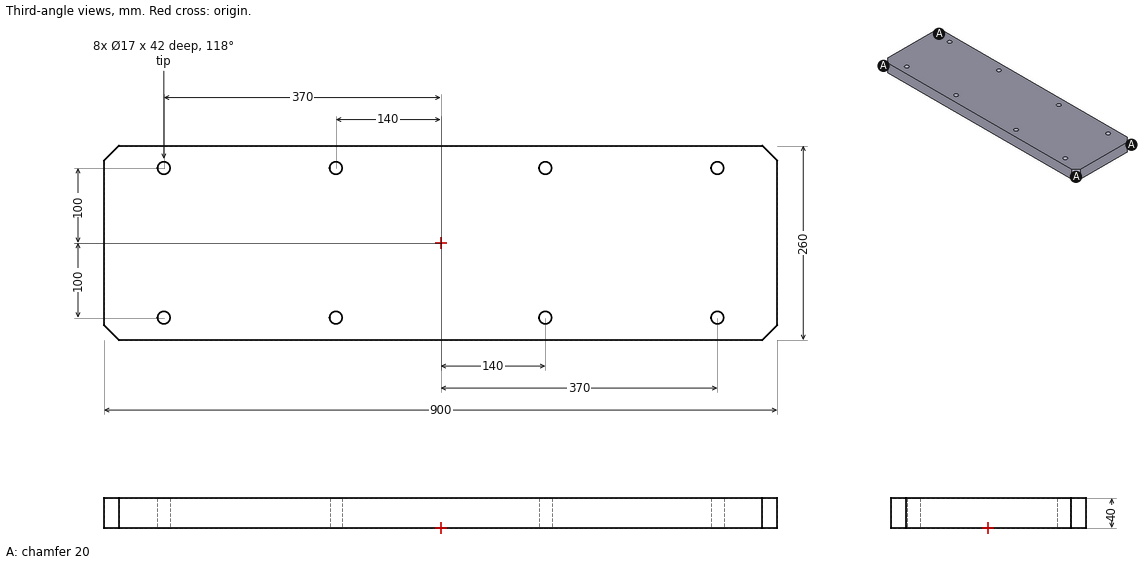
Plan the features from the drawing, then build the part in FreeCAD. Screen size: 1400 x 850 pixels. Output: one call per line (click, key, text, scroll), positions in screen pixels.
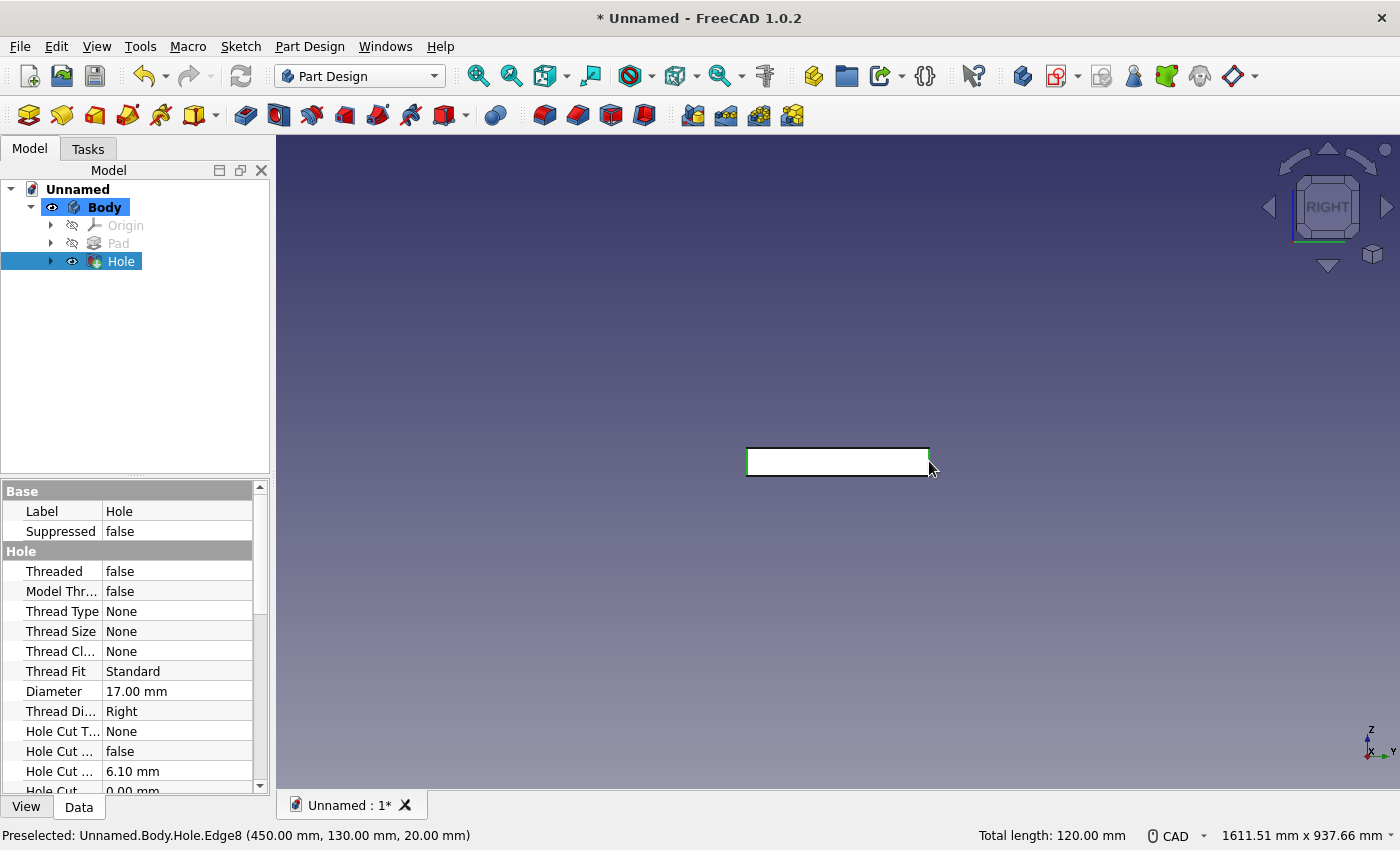
key(5)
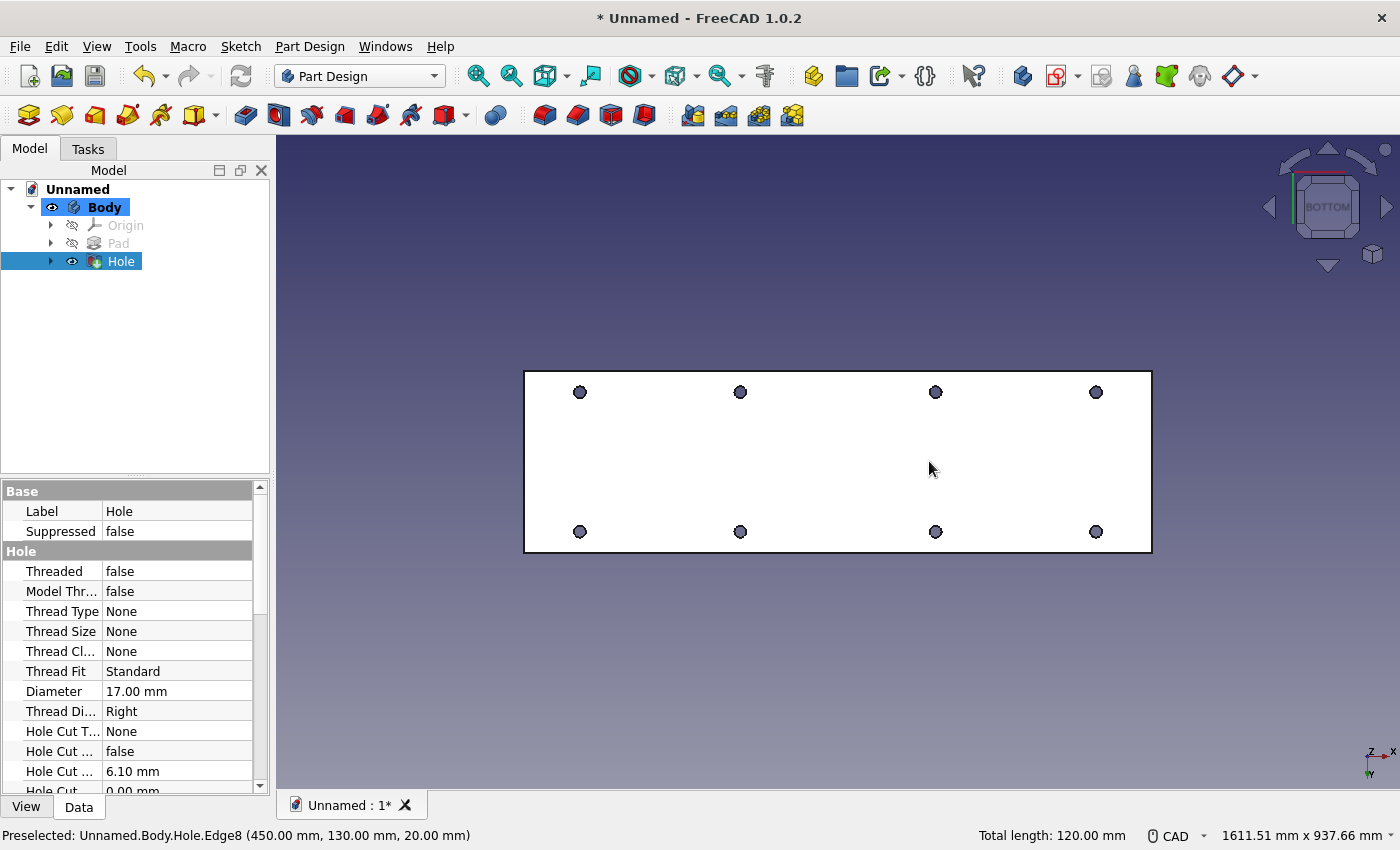
key(4)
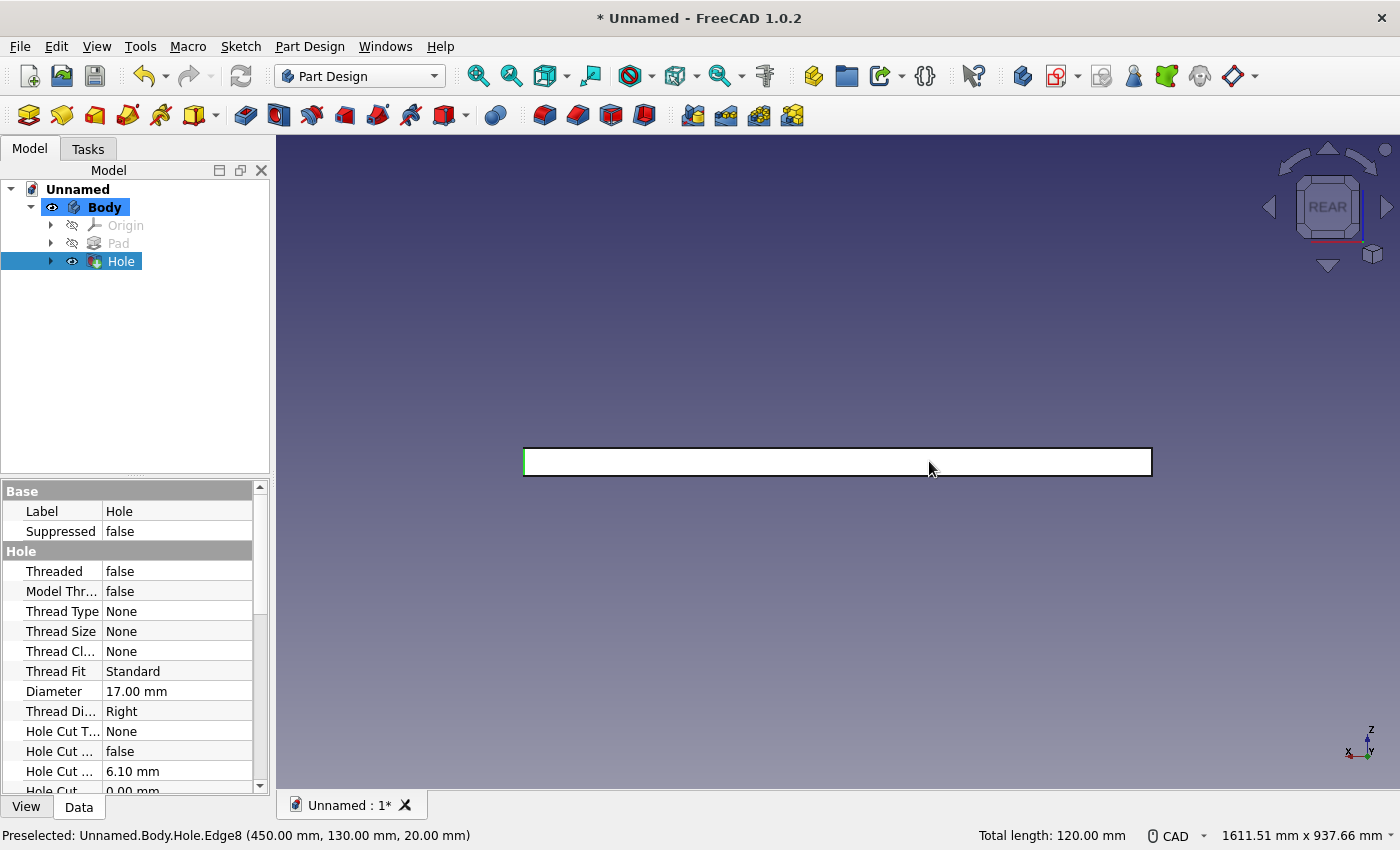
click(1152, 461, ctrl)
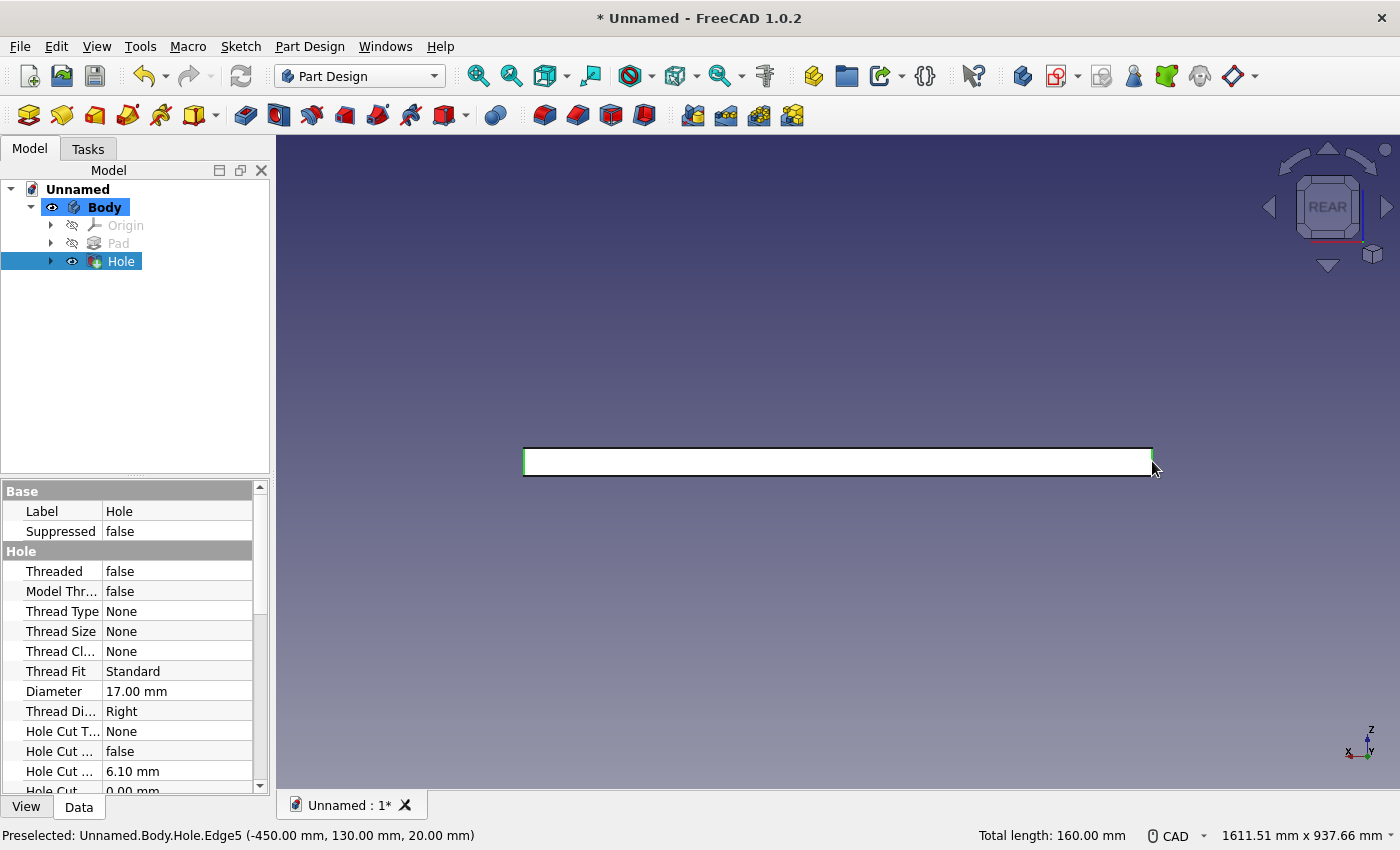
click(578, 116)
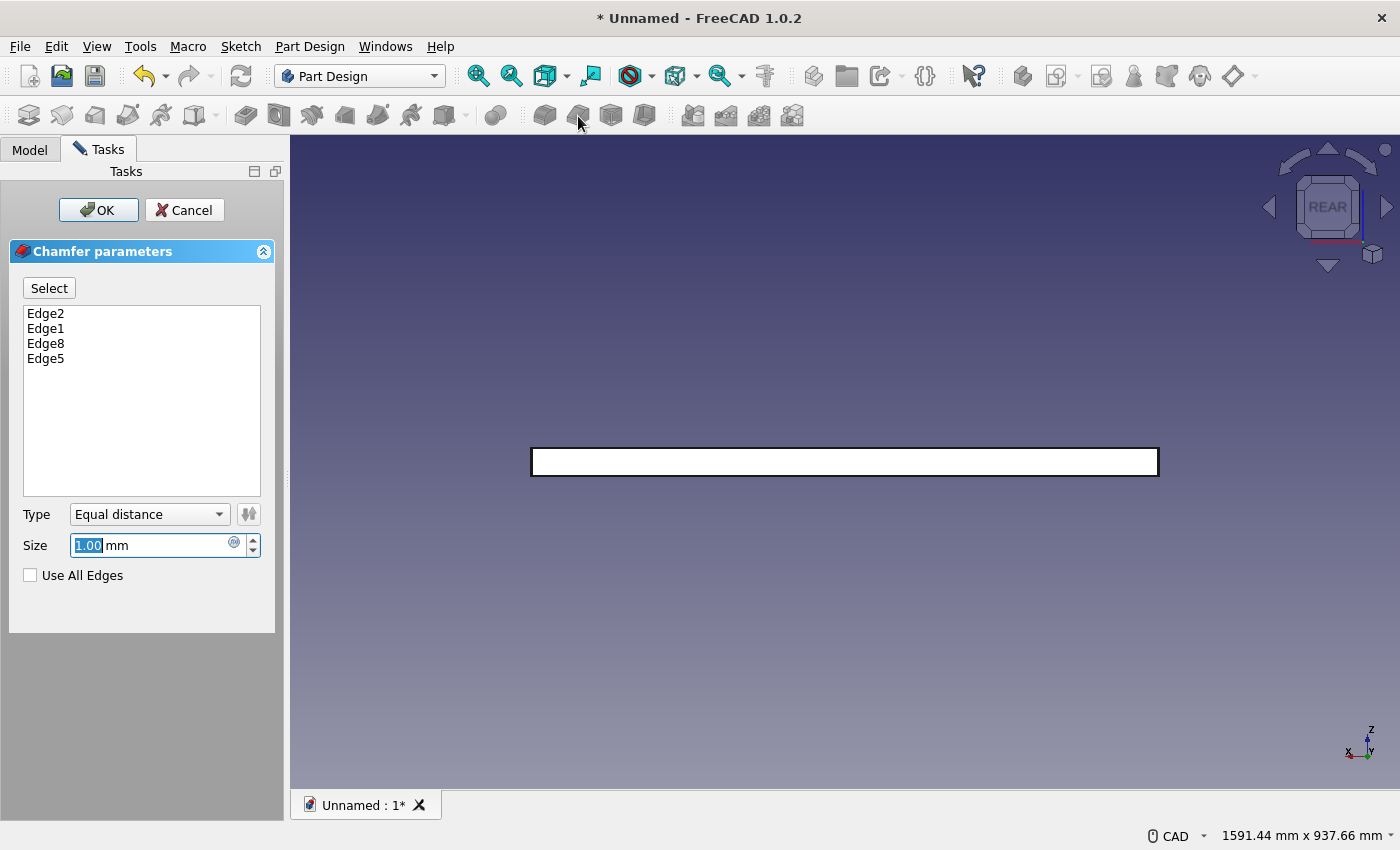
text(20)
key(Tab)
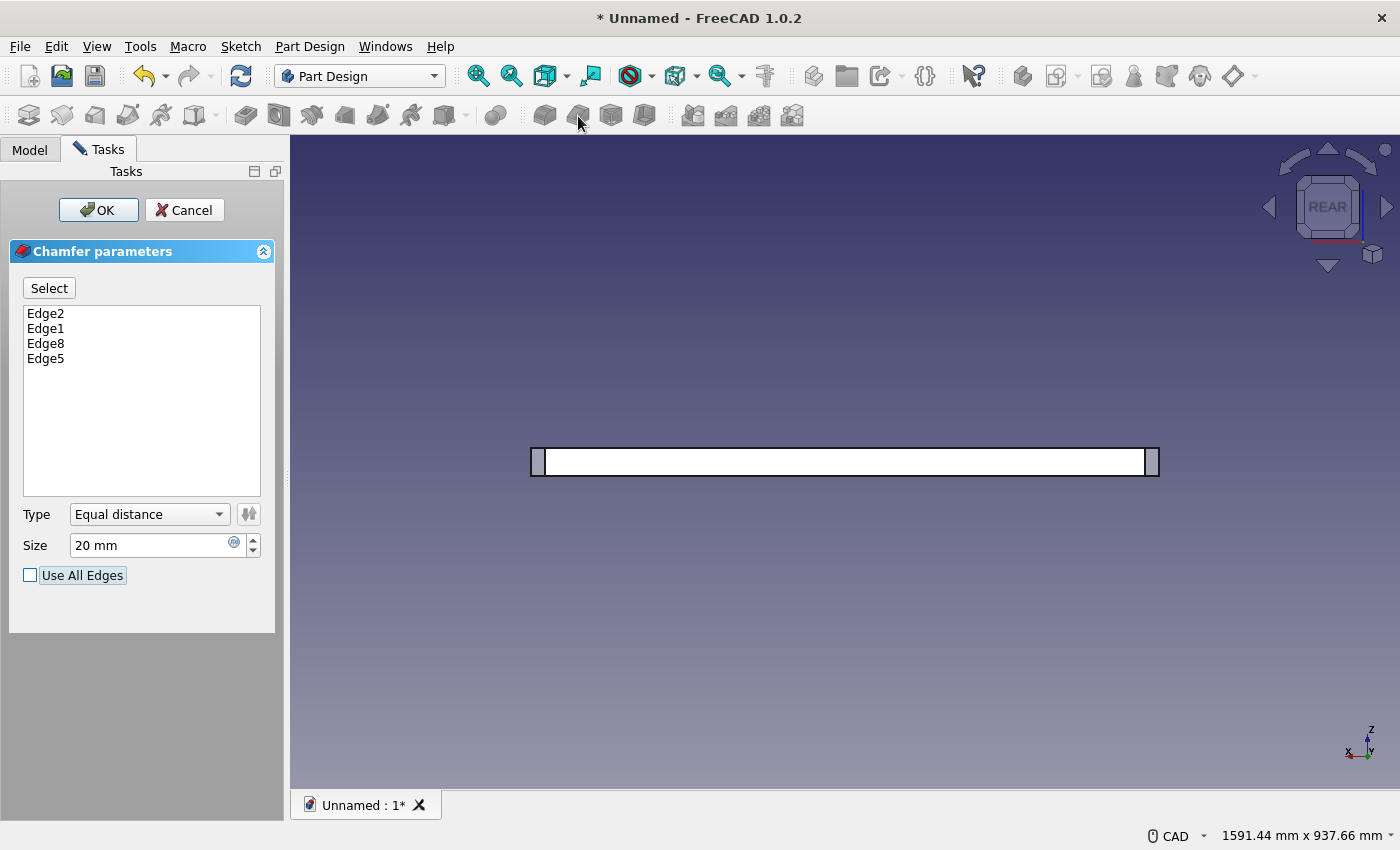
click(99, 210)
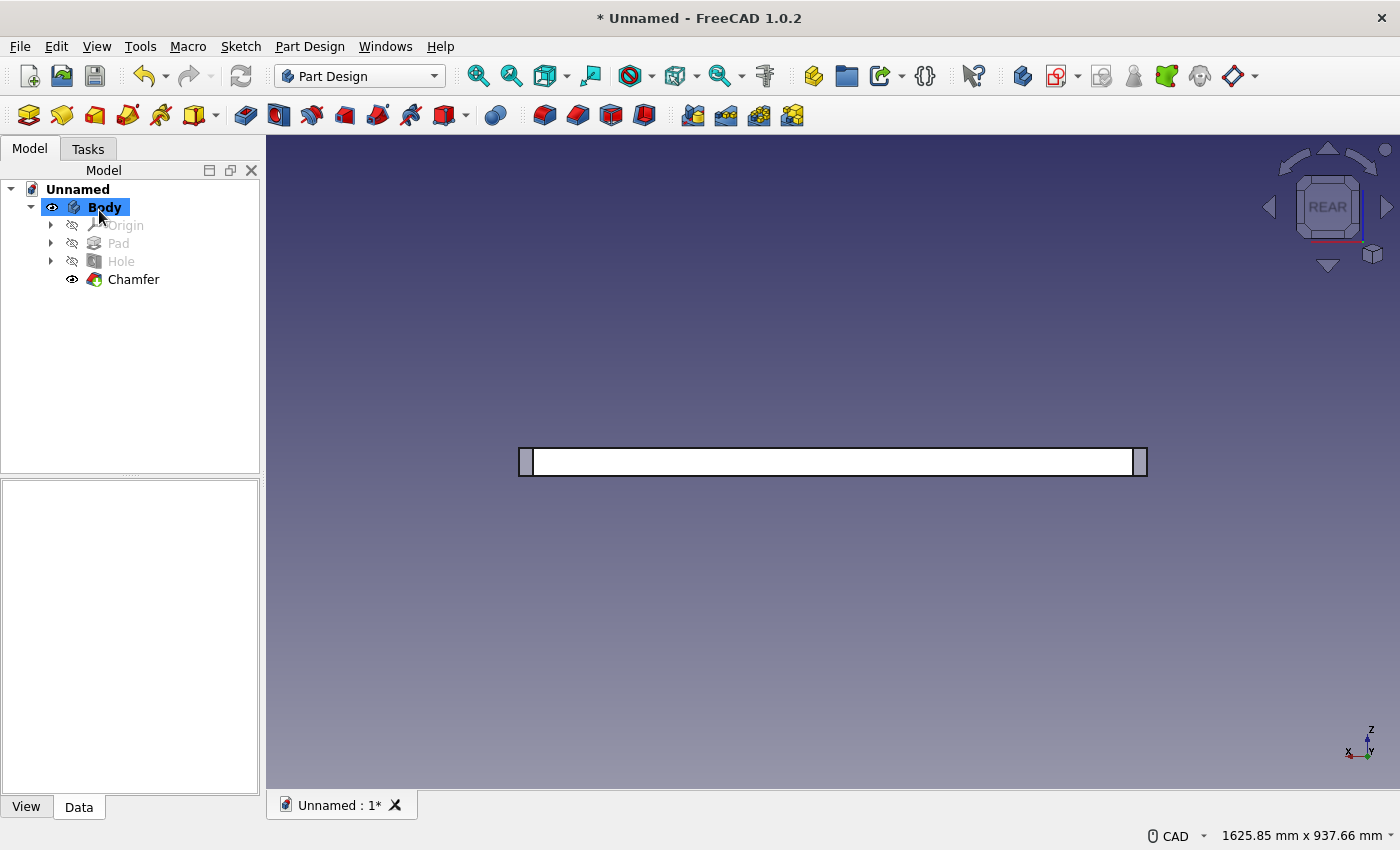
key(0)